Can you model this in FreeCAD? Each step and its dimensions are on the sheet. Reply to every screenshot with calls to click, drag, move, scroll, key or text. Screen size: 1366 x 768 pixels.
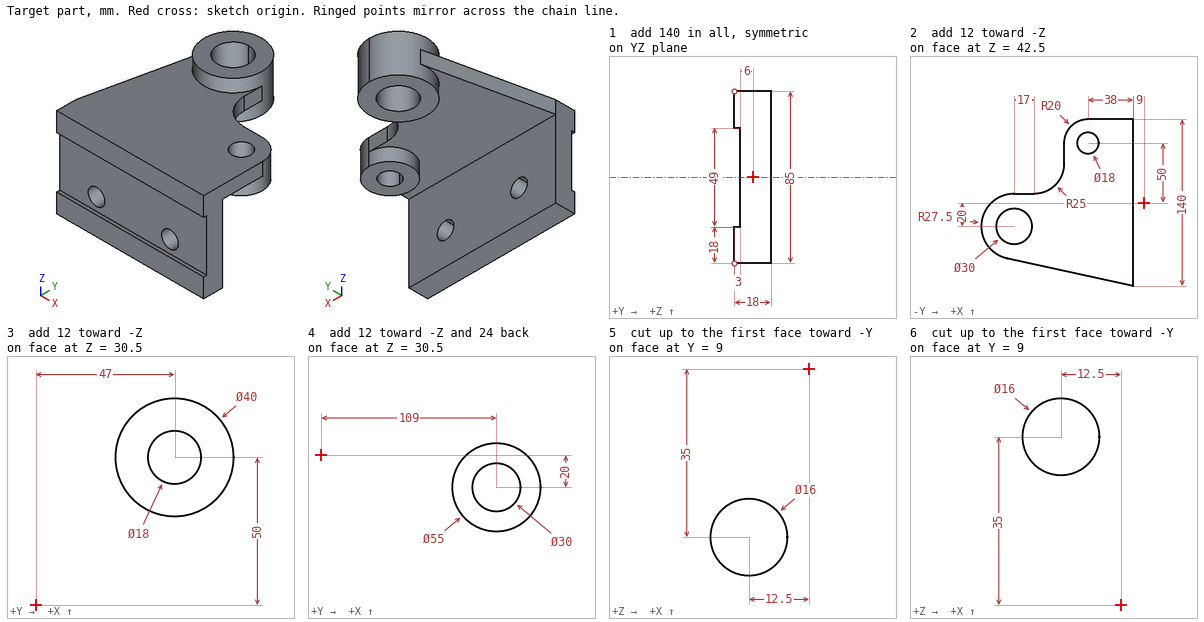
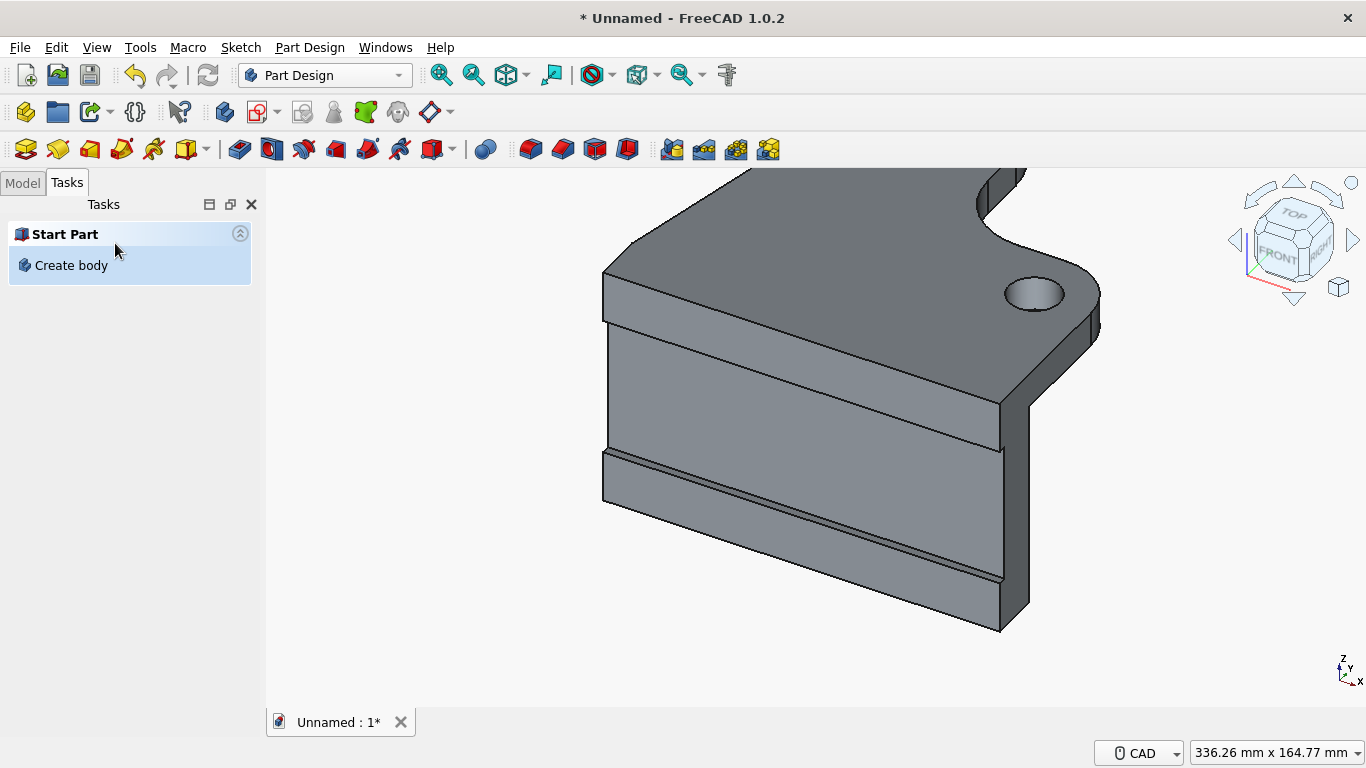
key(v)
key(f)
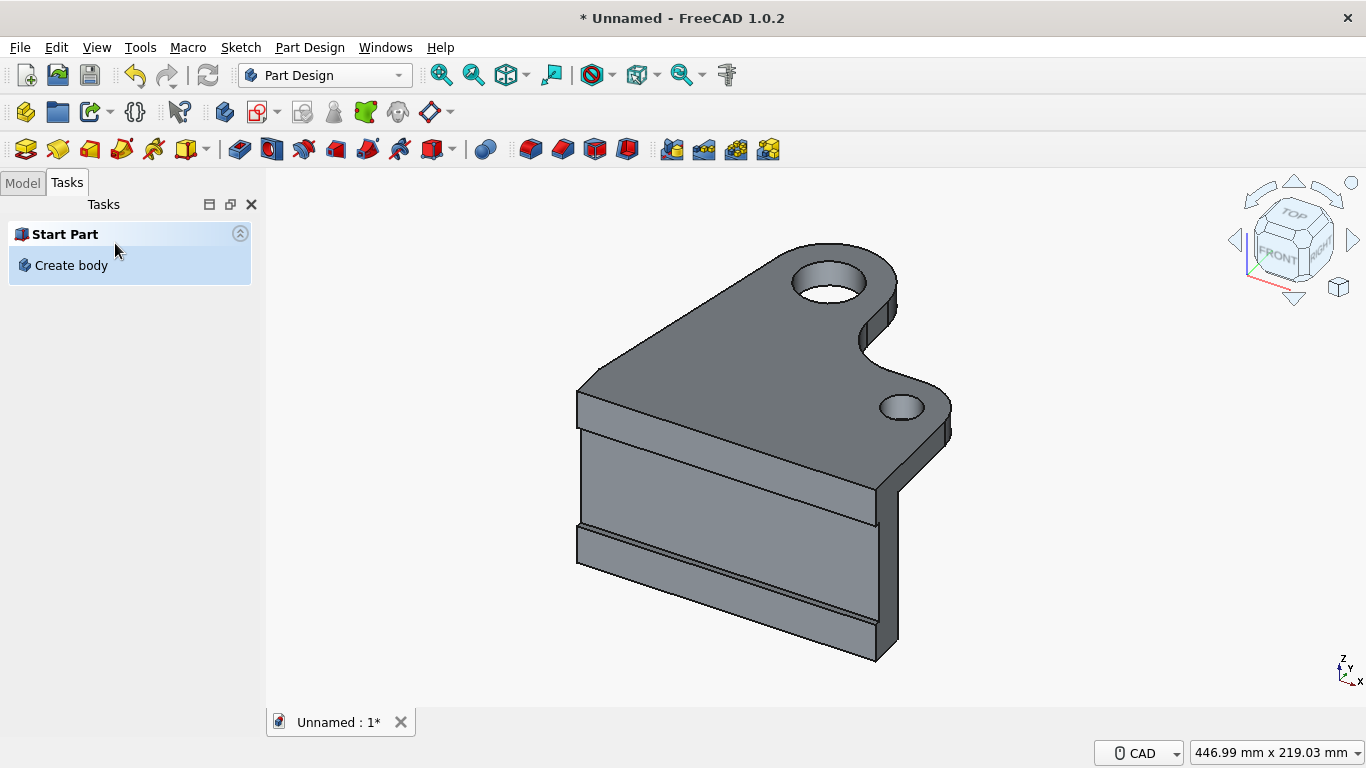
key(5)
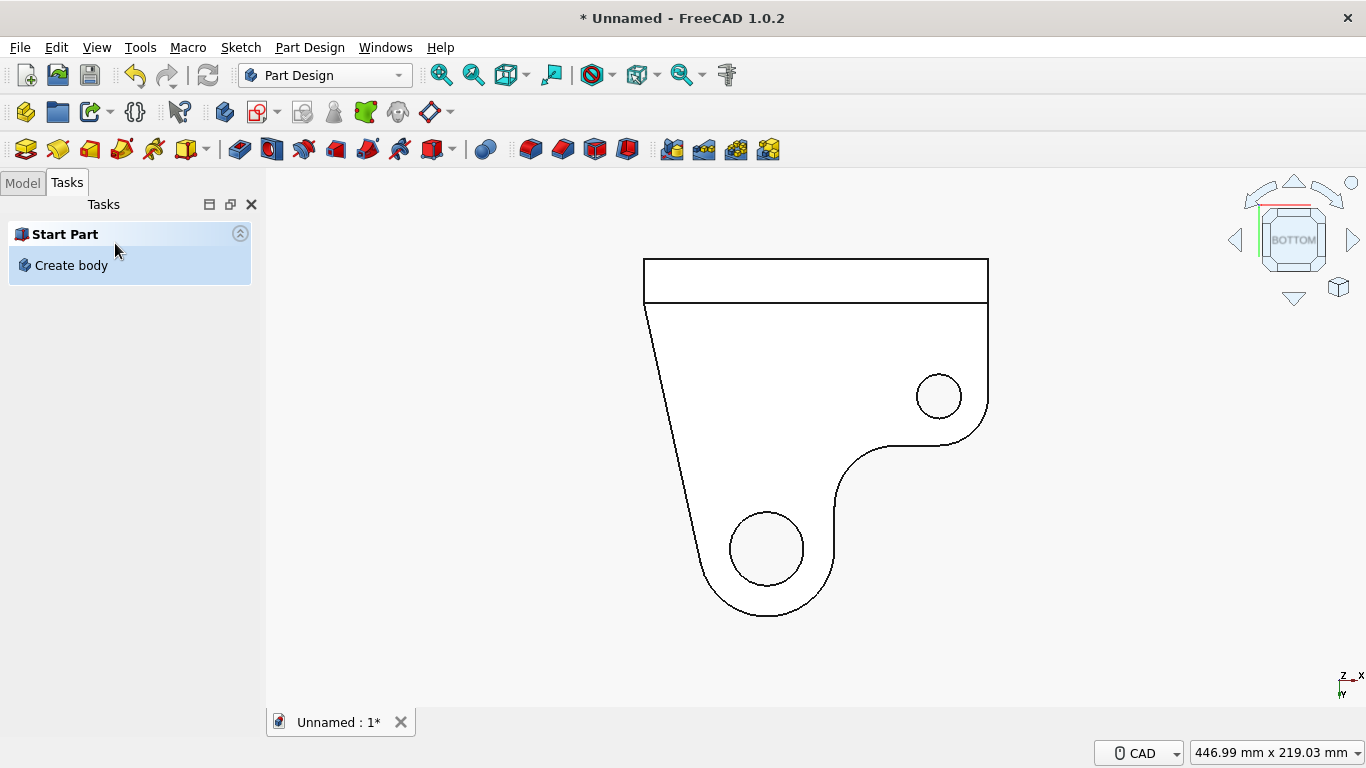
click(767, 414)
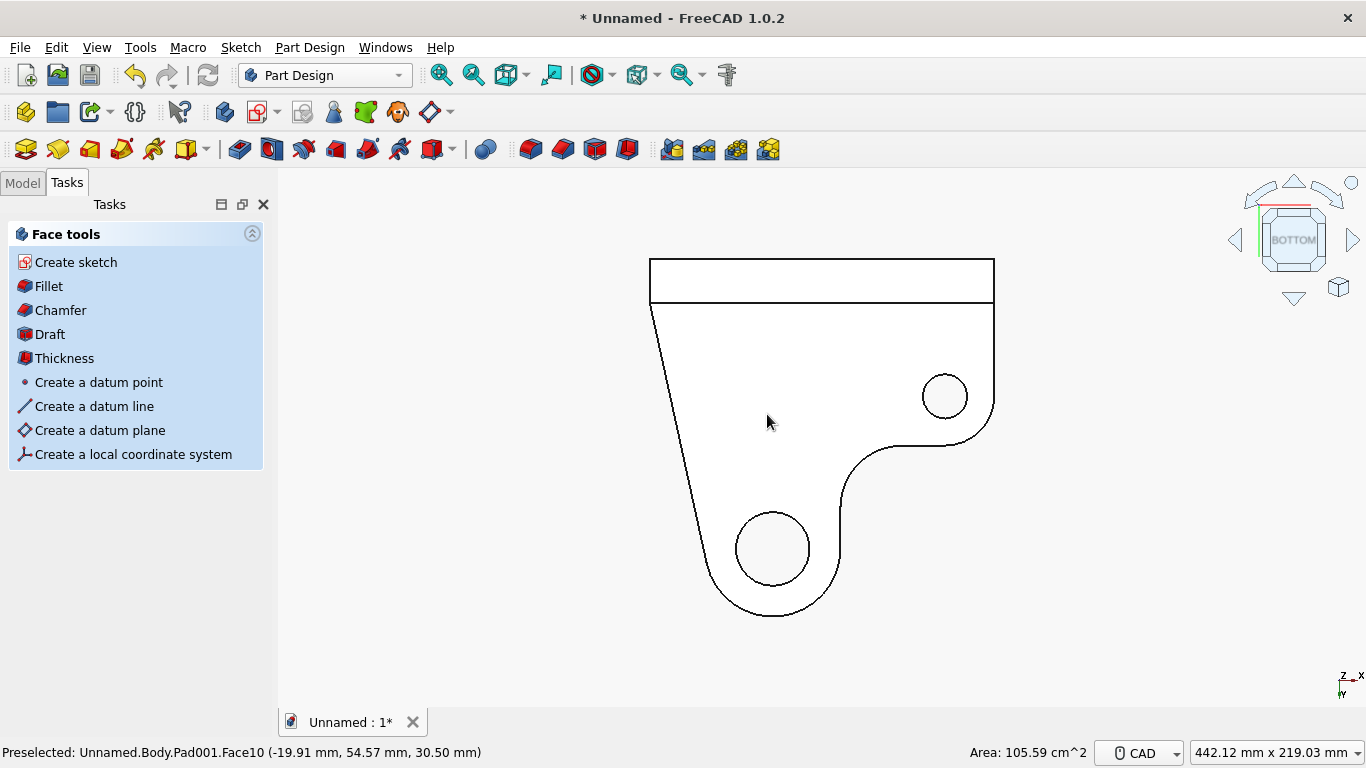
click(258, 112)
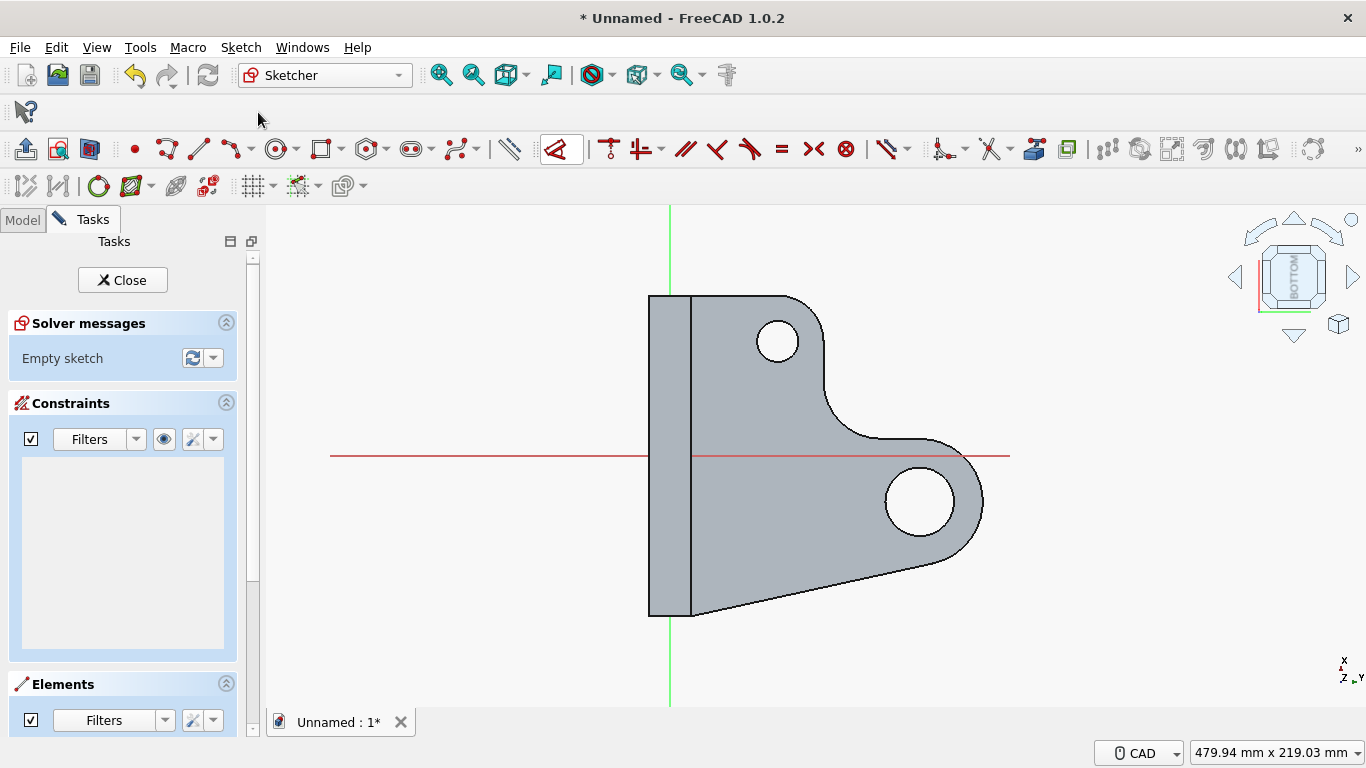
key(q)
key(s)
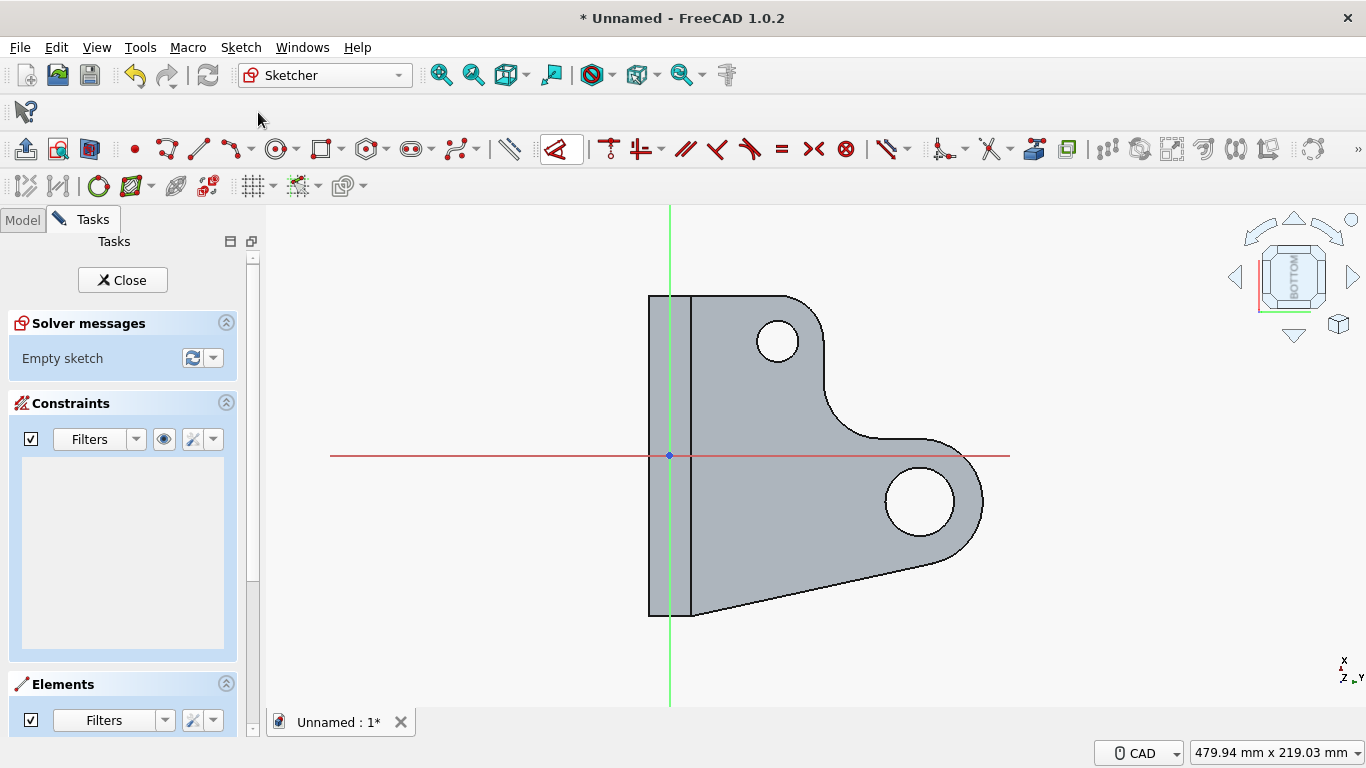
scroll(746, 278, up, 3)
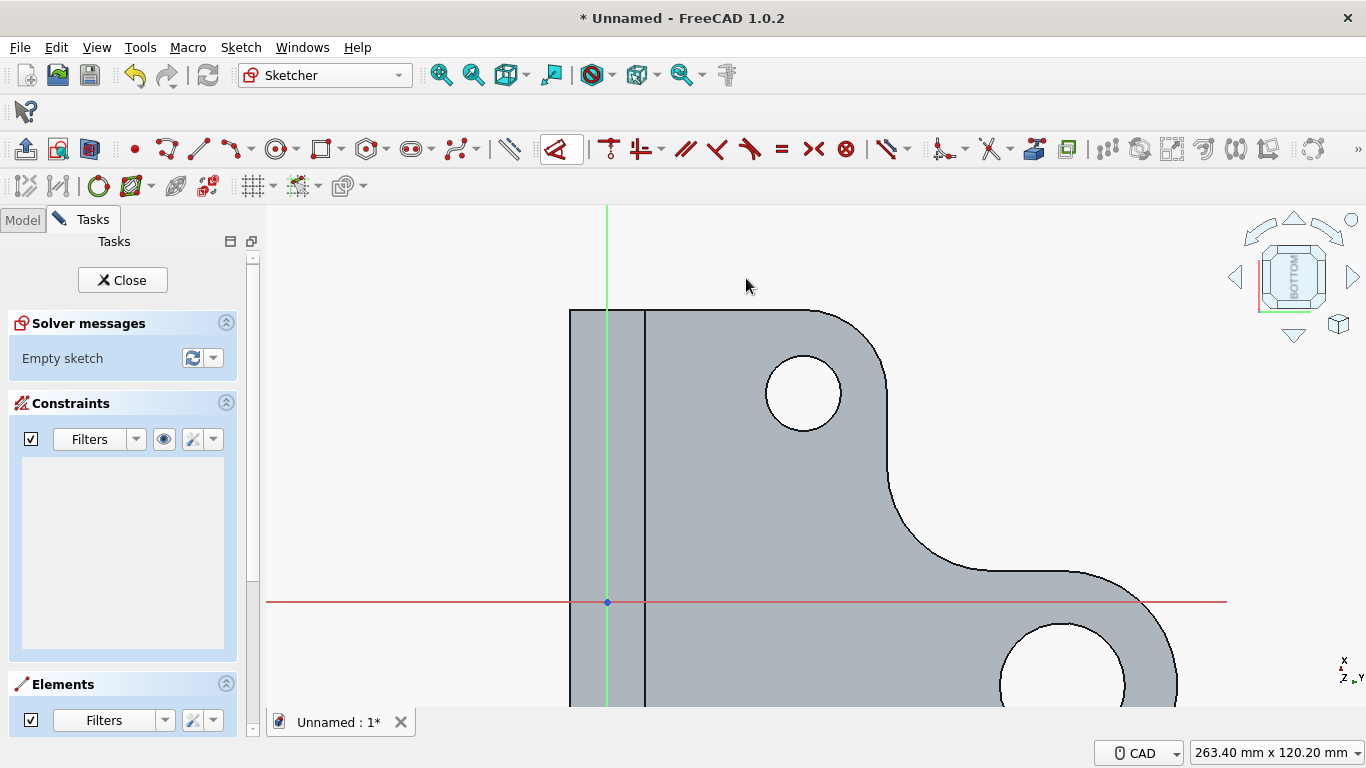
key(g)
key(c)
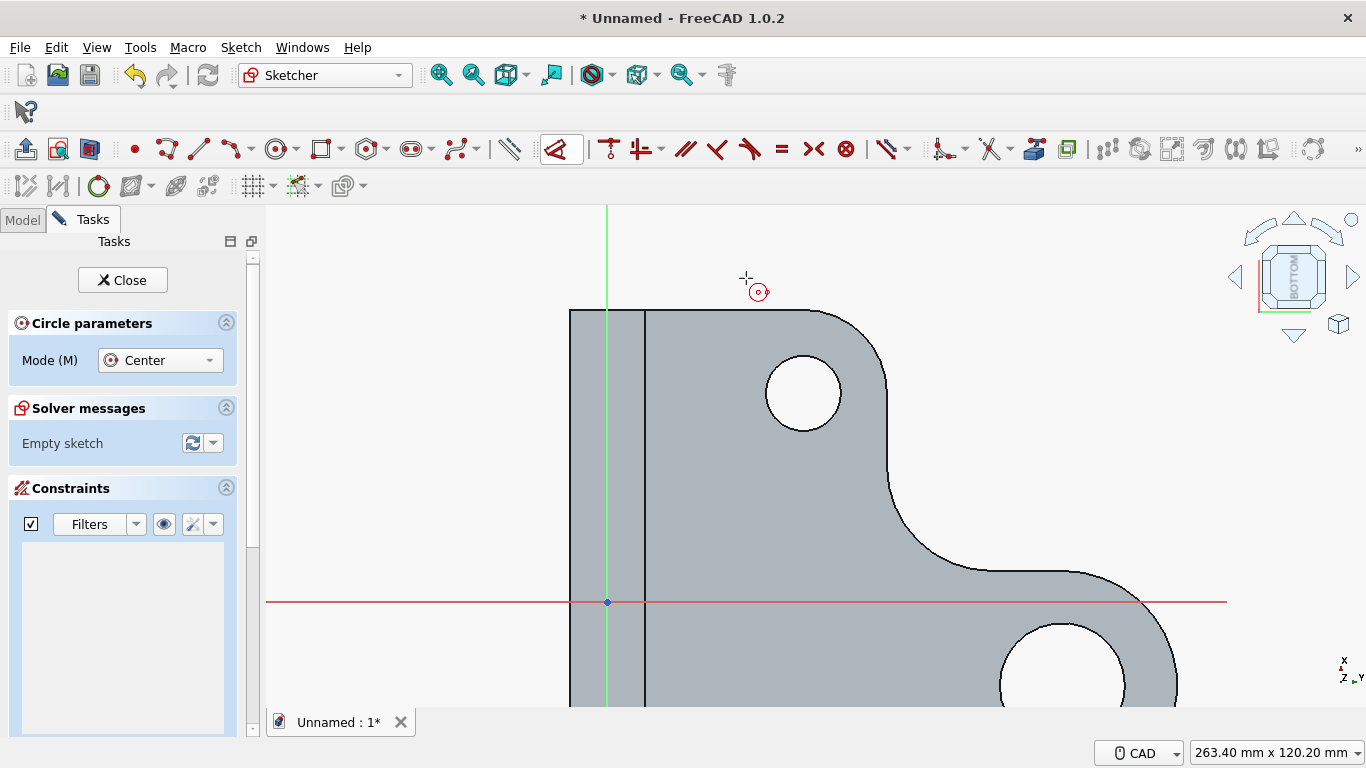
click(803, 393)
move(862, 334)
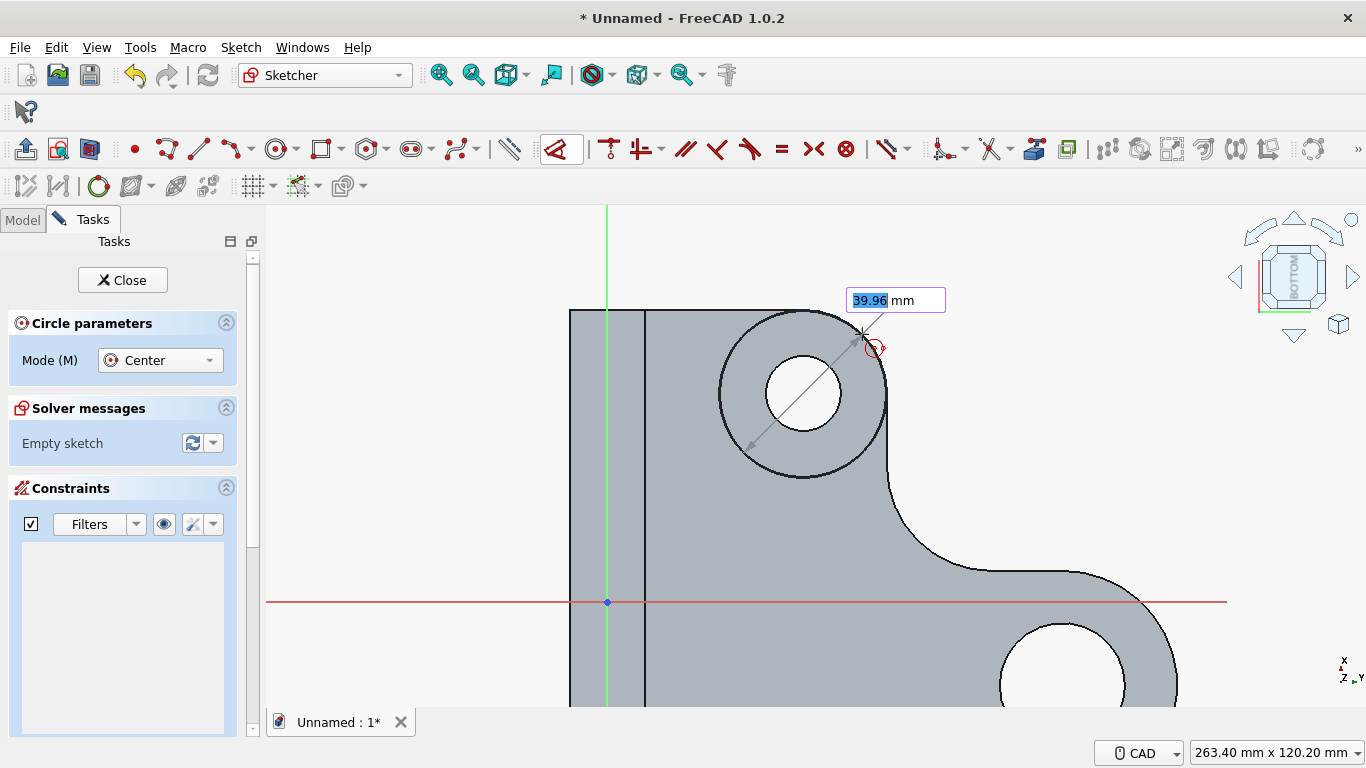
text(40)
key(Return)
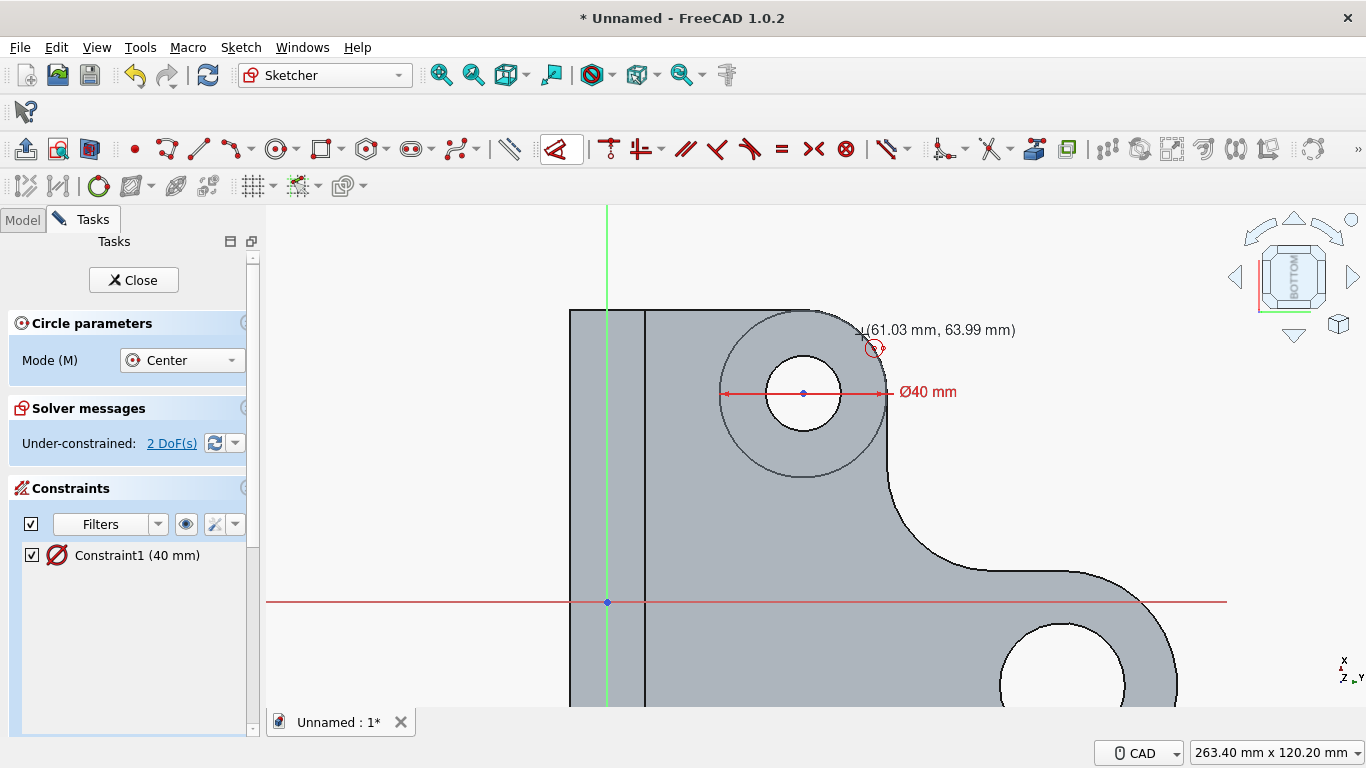
click(803, 394)
move(830, 367)